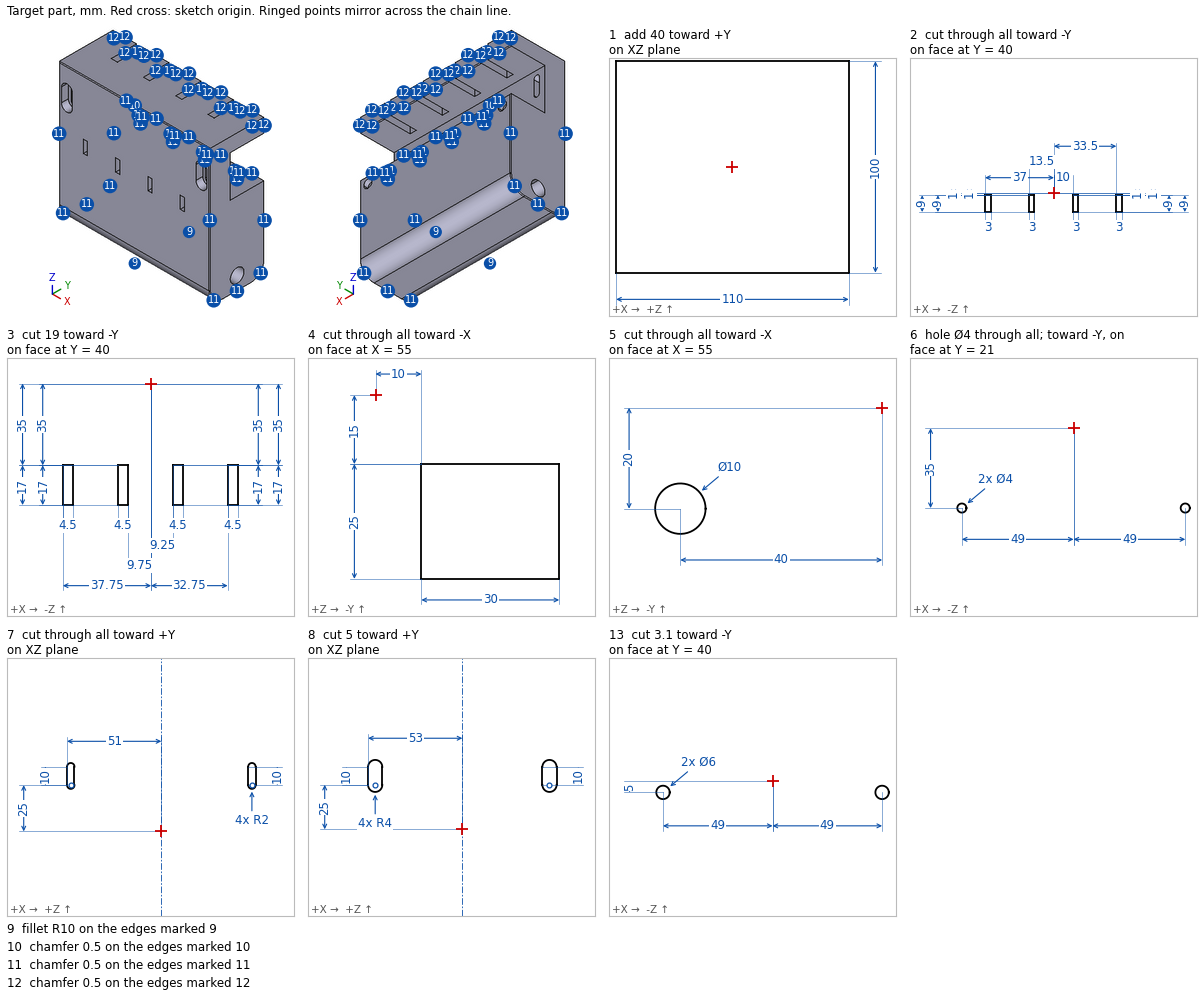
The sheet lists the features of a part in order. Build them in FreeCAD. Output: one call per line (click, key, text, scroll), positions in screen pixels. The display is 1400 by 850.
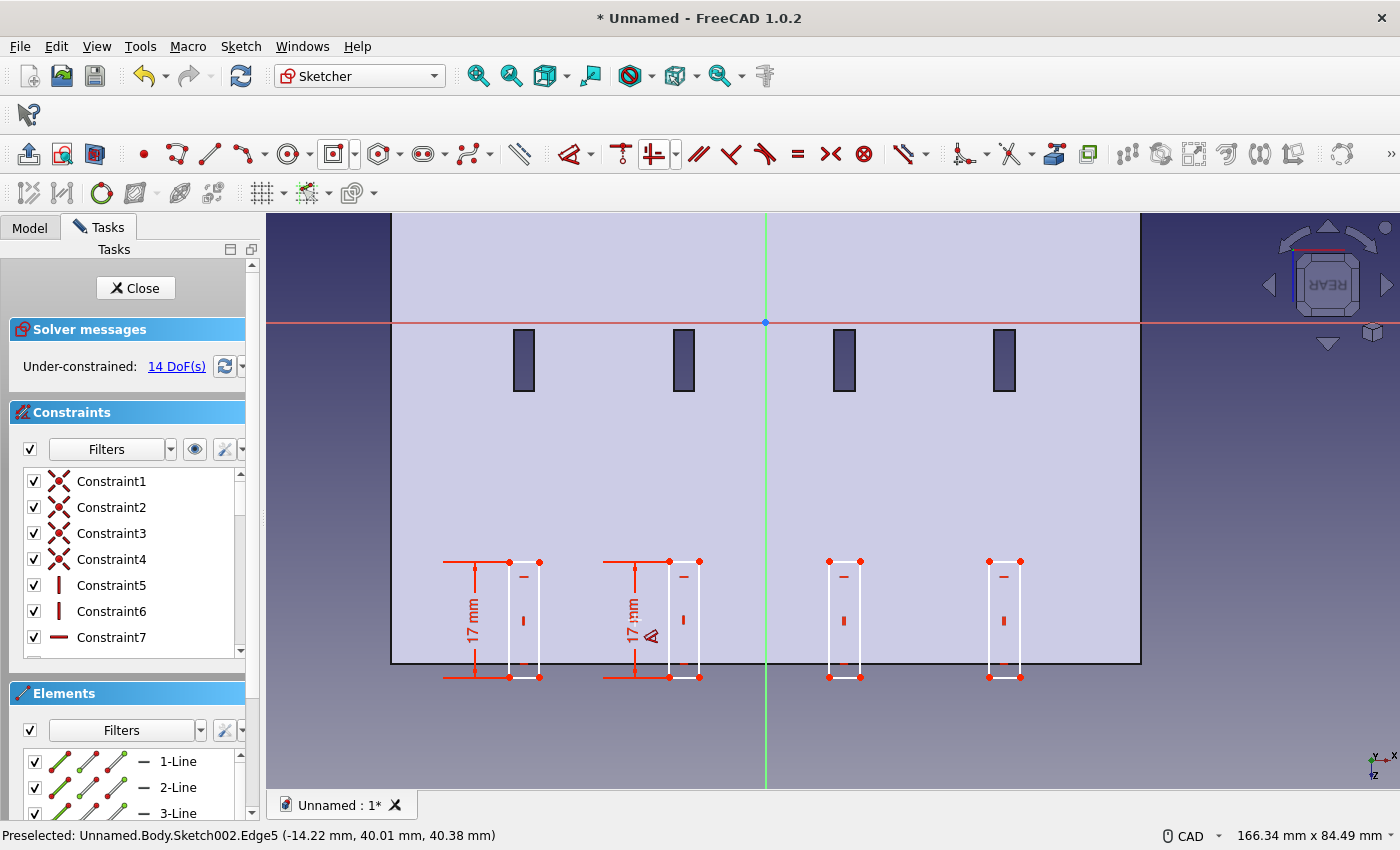
click(829, 597)
click(795, 620)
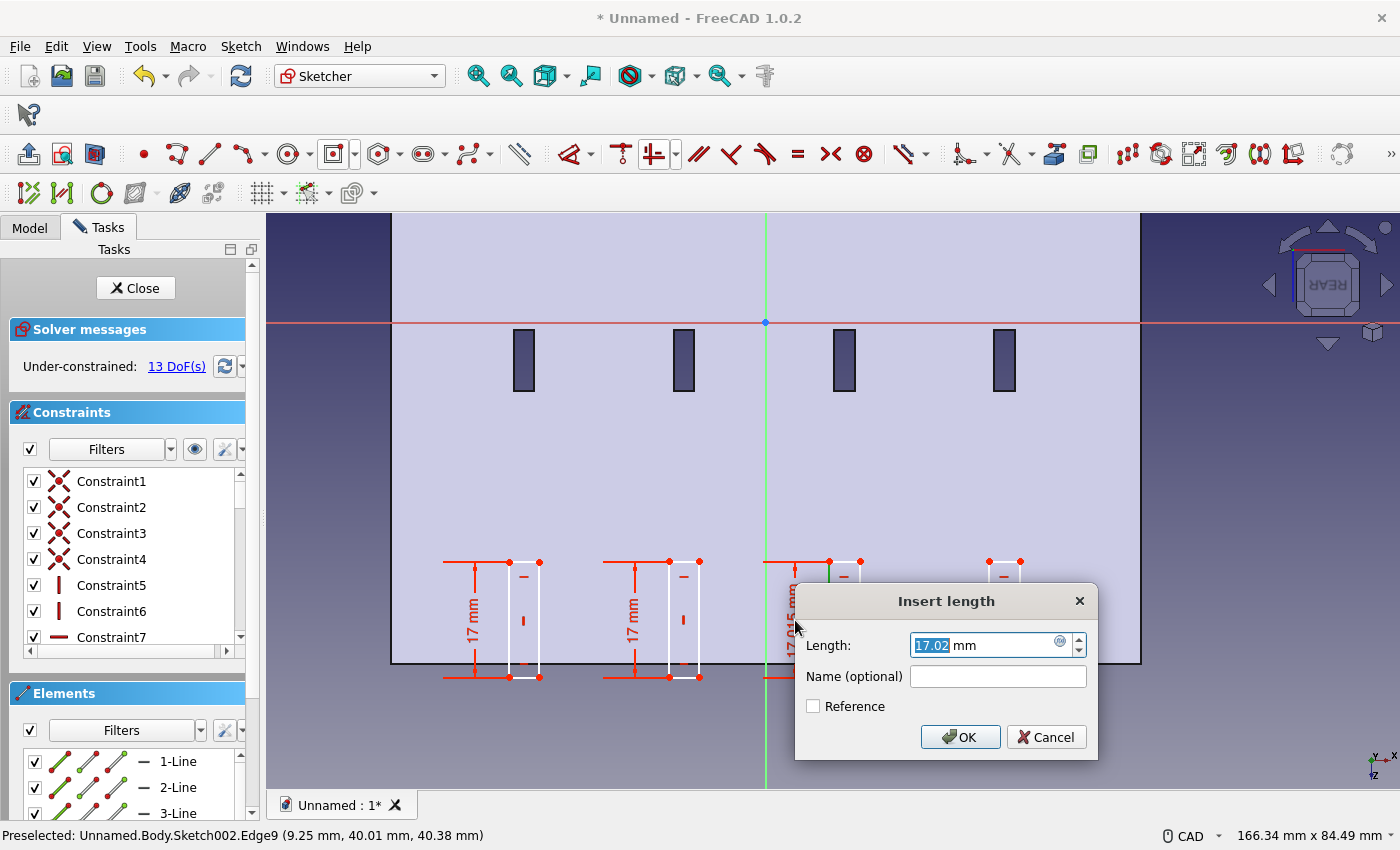
text(17)
key(Return)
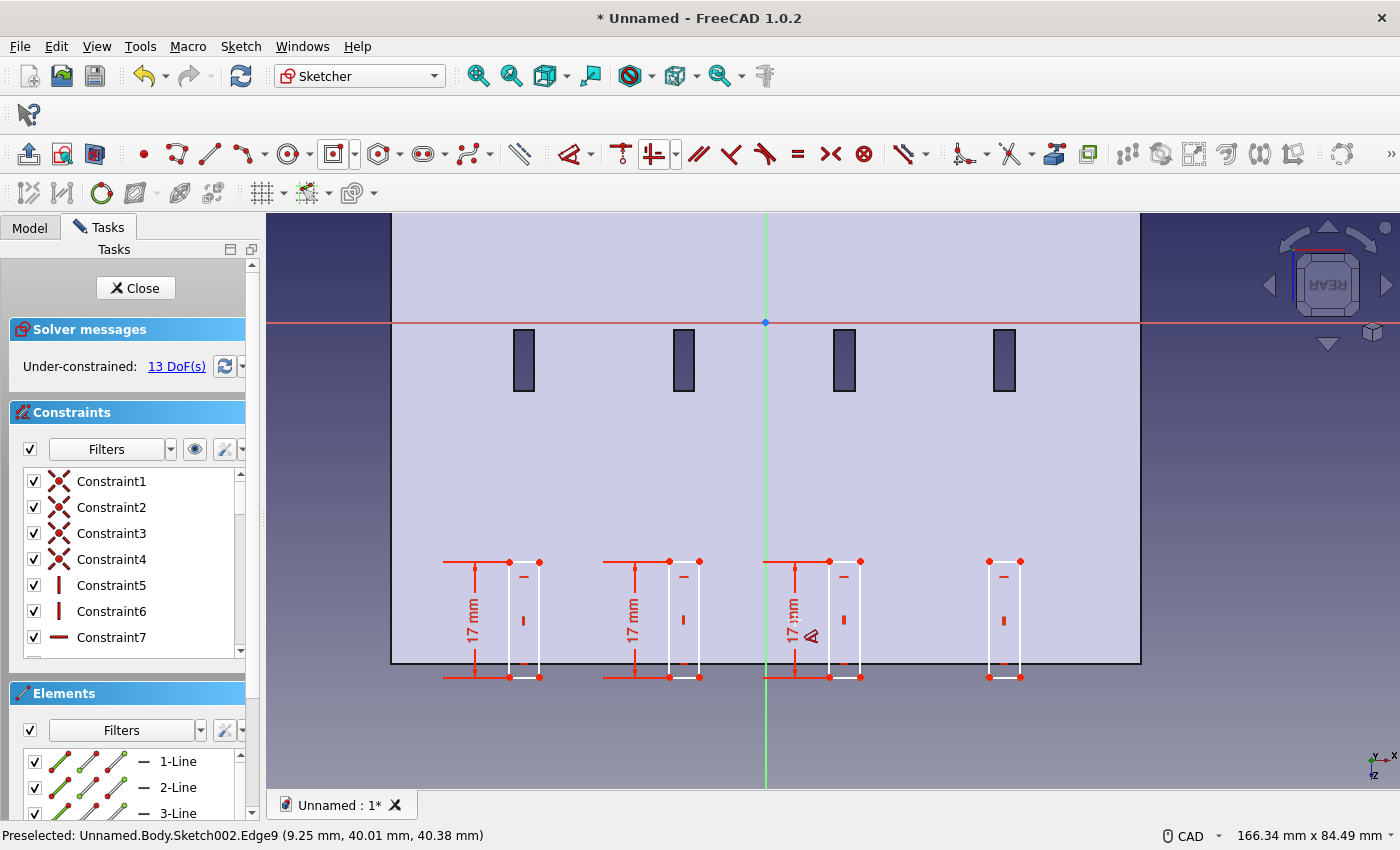
click(989, 597)
click(955, 620)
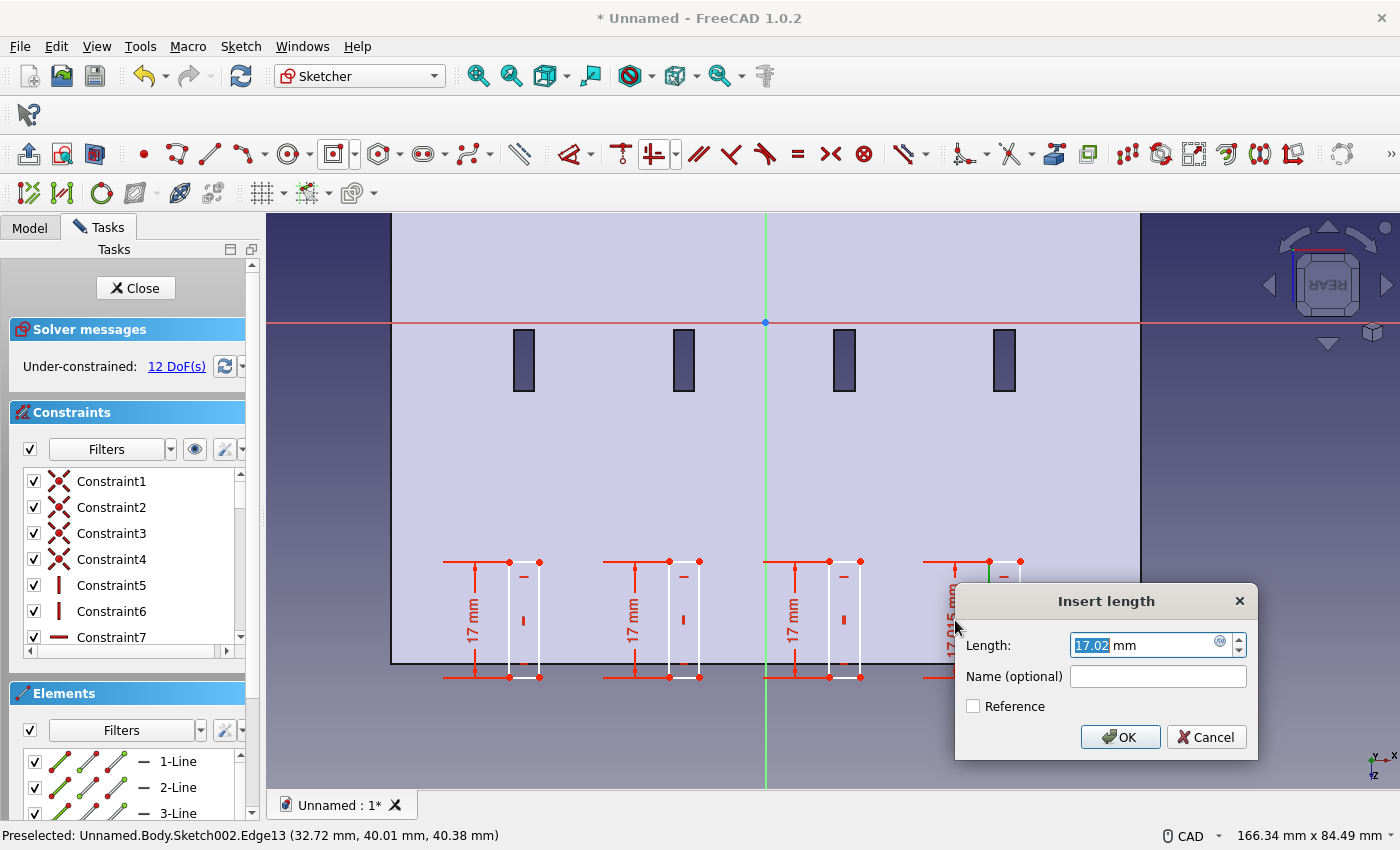
text(17)
key(Return)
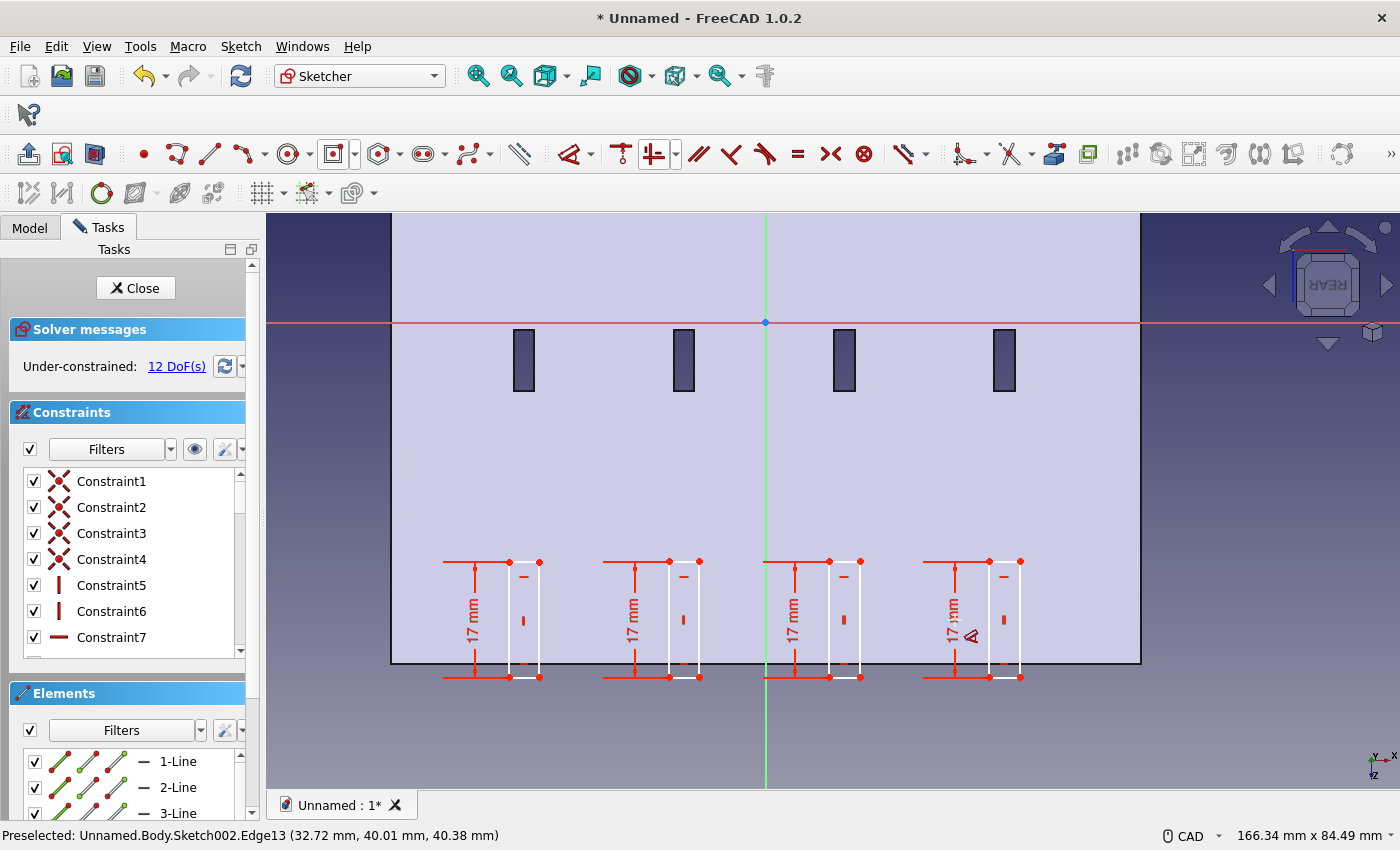
scroll(521, 678, up, 2)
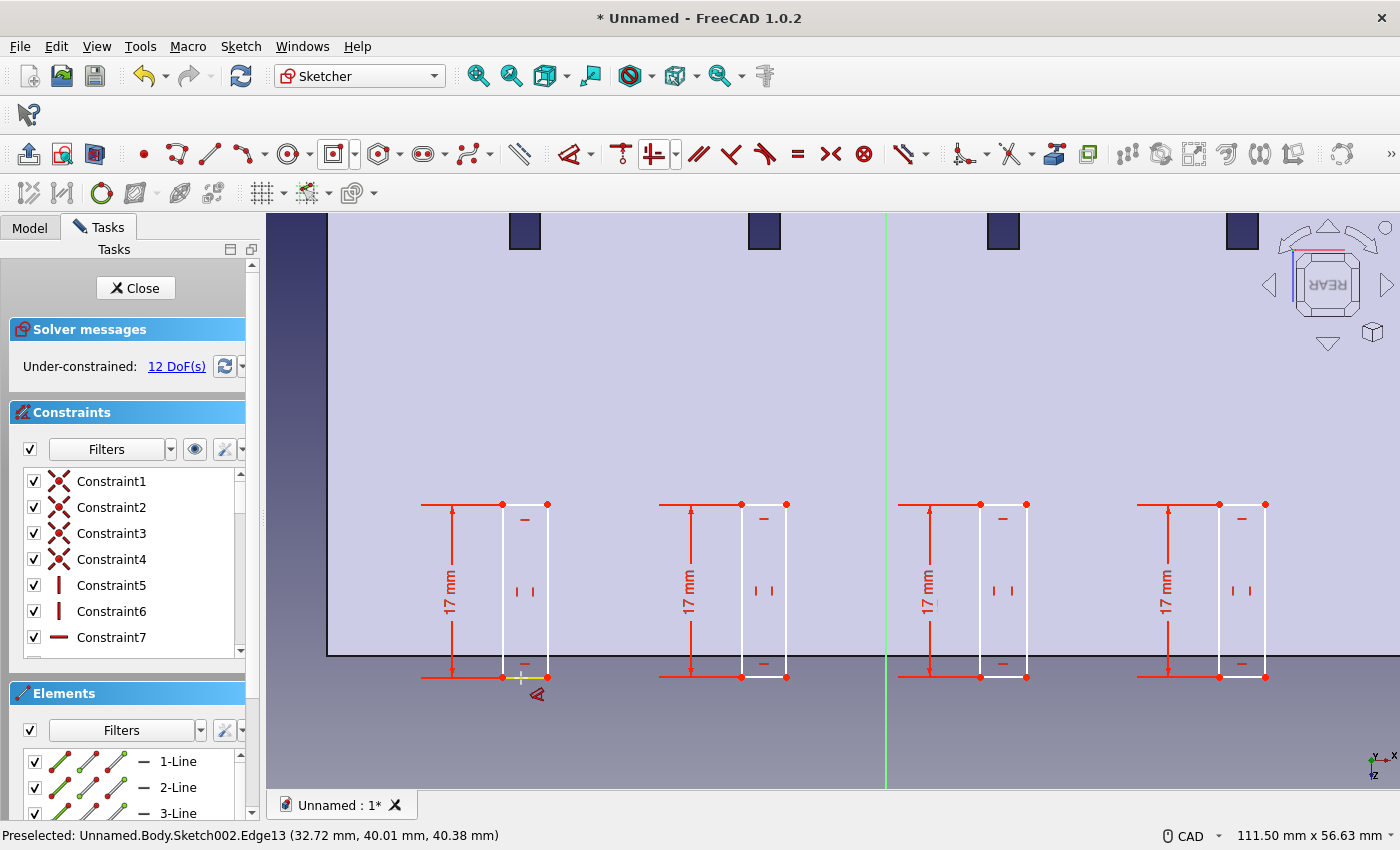
click(521, 678)
click(525, 712)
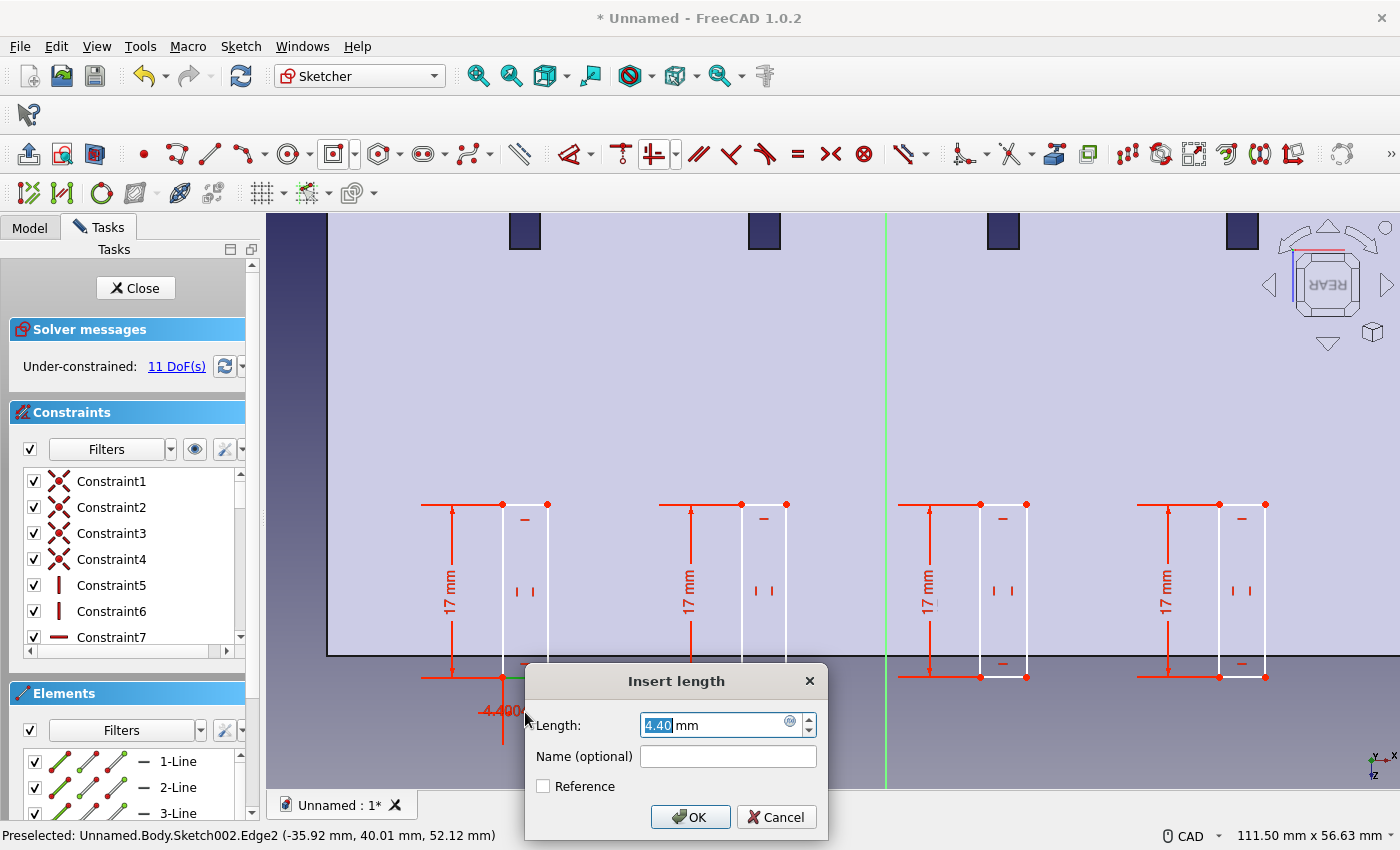
text(4.5)
key(Return)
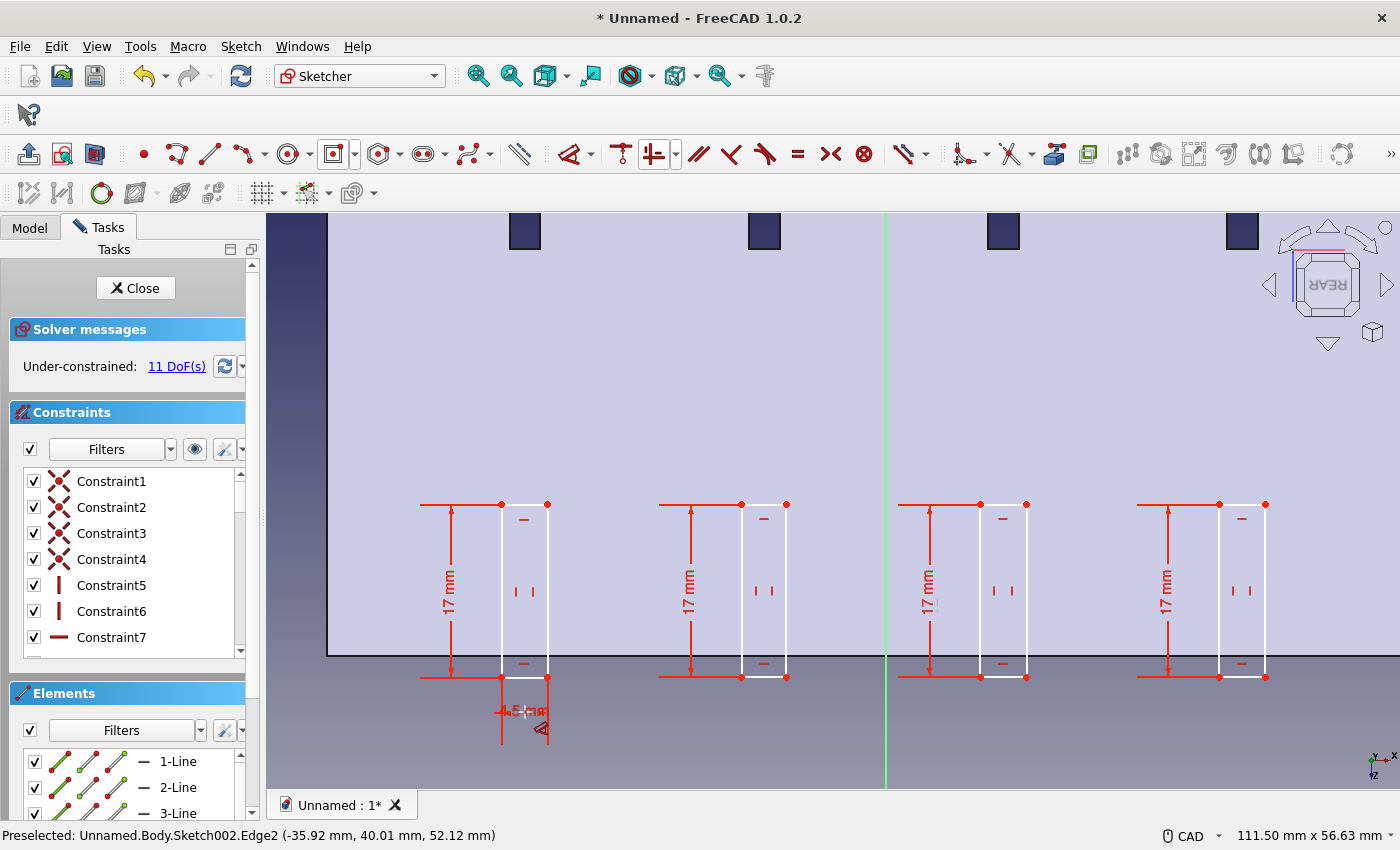
click(755, 677)
click(764, 711)